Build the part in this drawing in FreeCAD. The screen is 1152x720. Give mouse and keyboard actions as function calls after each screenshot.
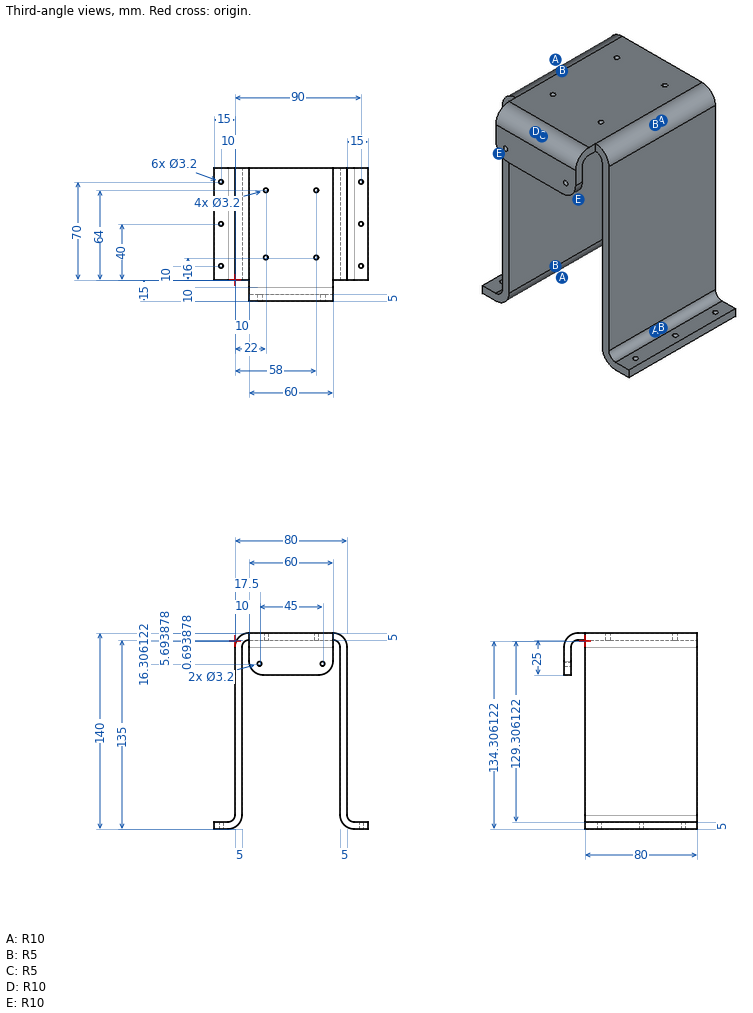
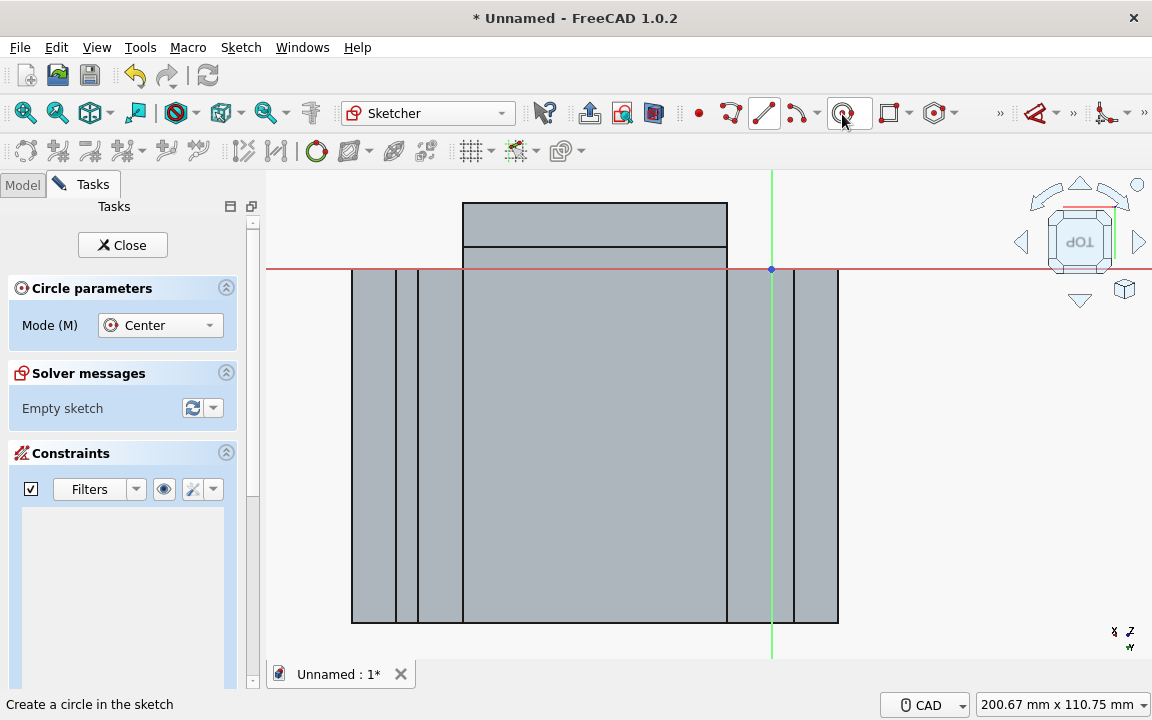
scroll(674, 552, up, 6)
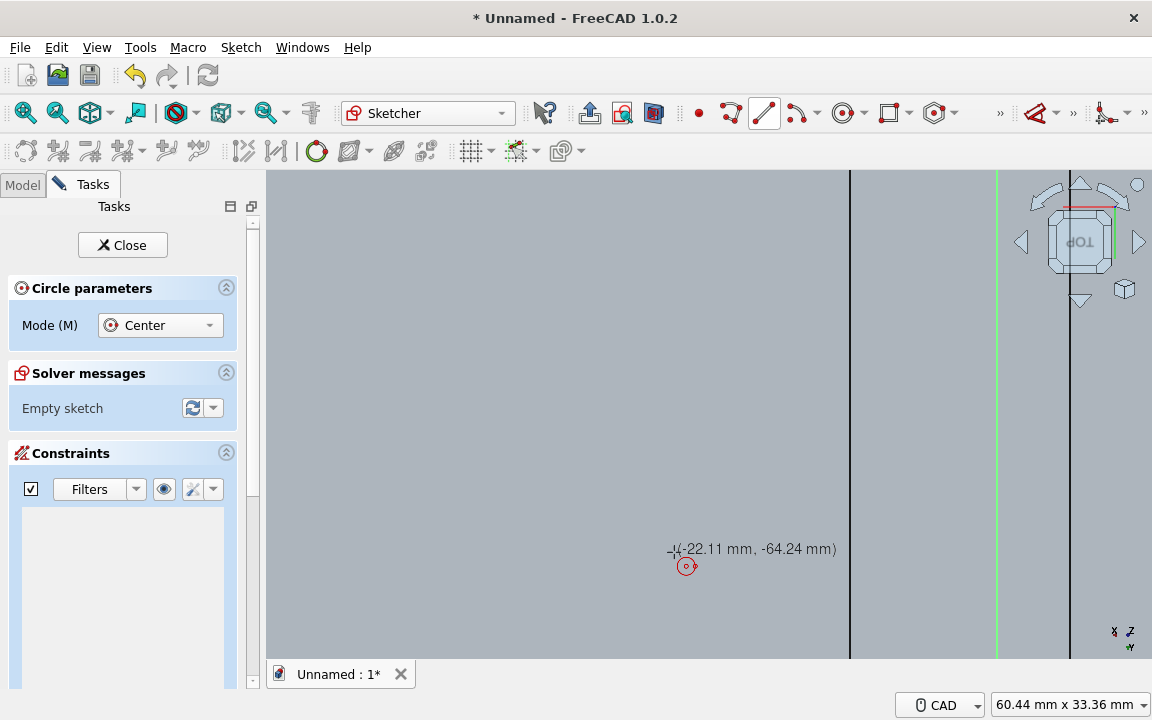
click(675, 550)
move(691, 533)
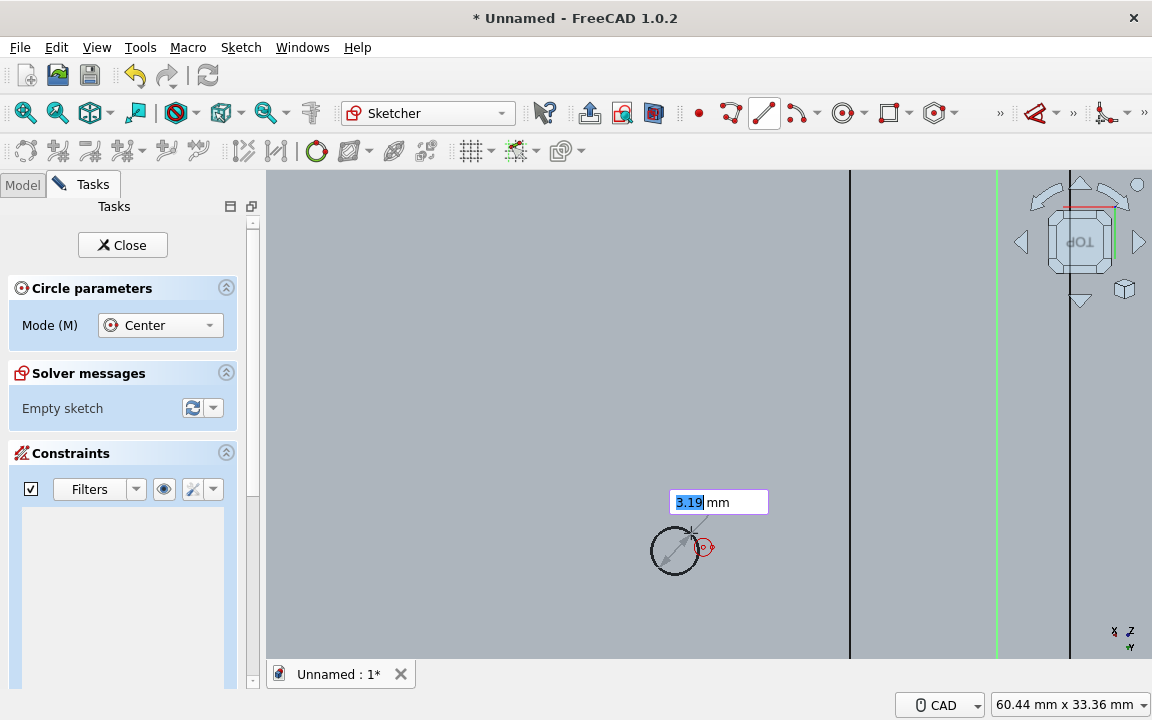
text(3.2)
key(Return)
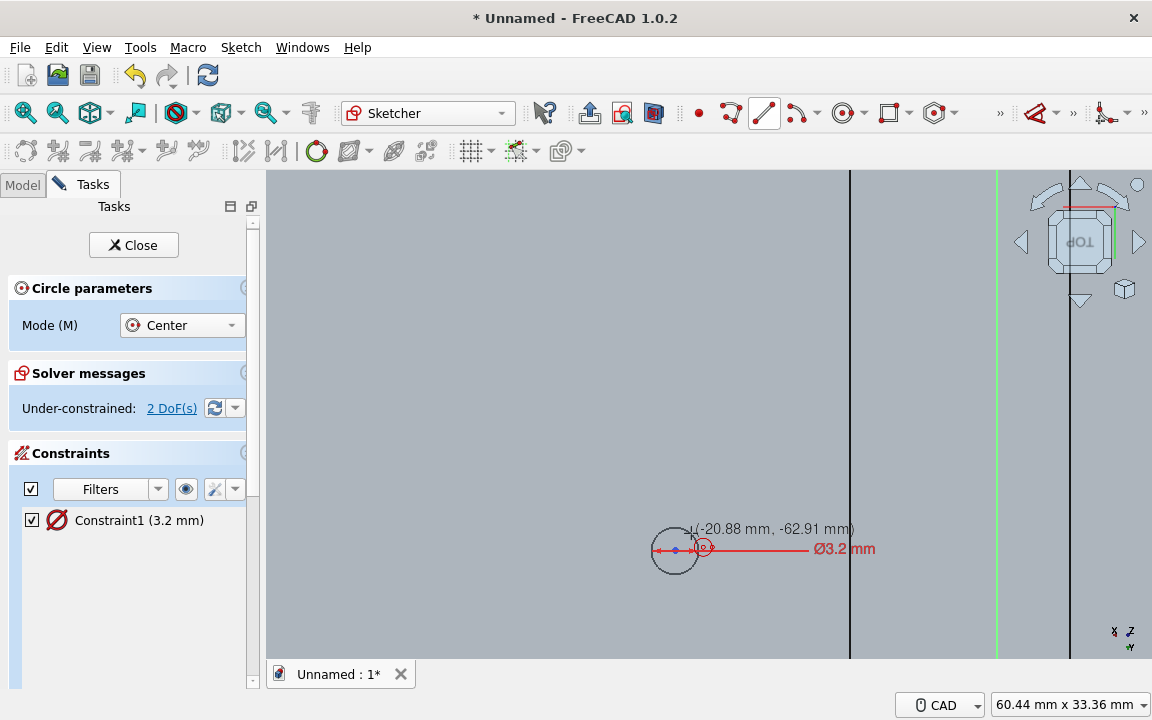
scroll(675, 553, down, 6)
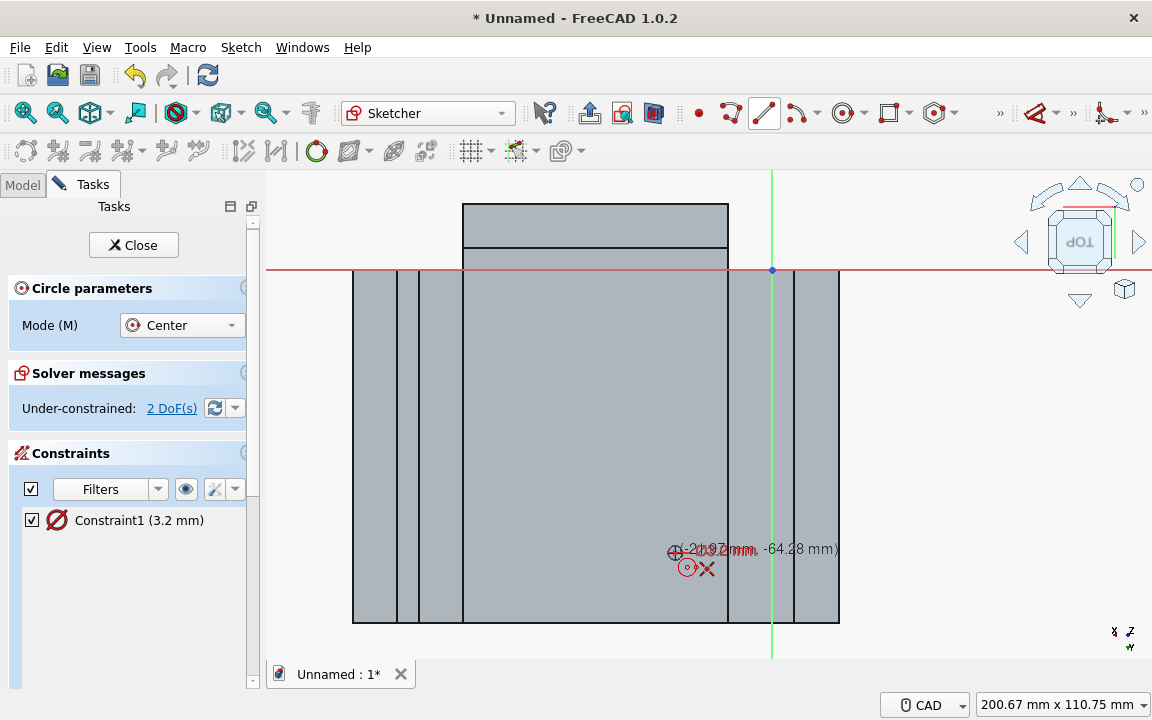
scroll(516, 553, up, 6)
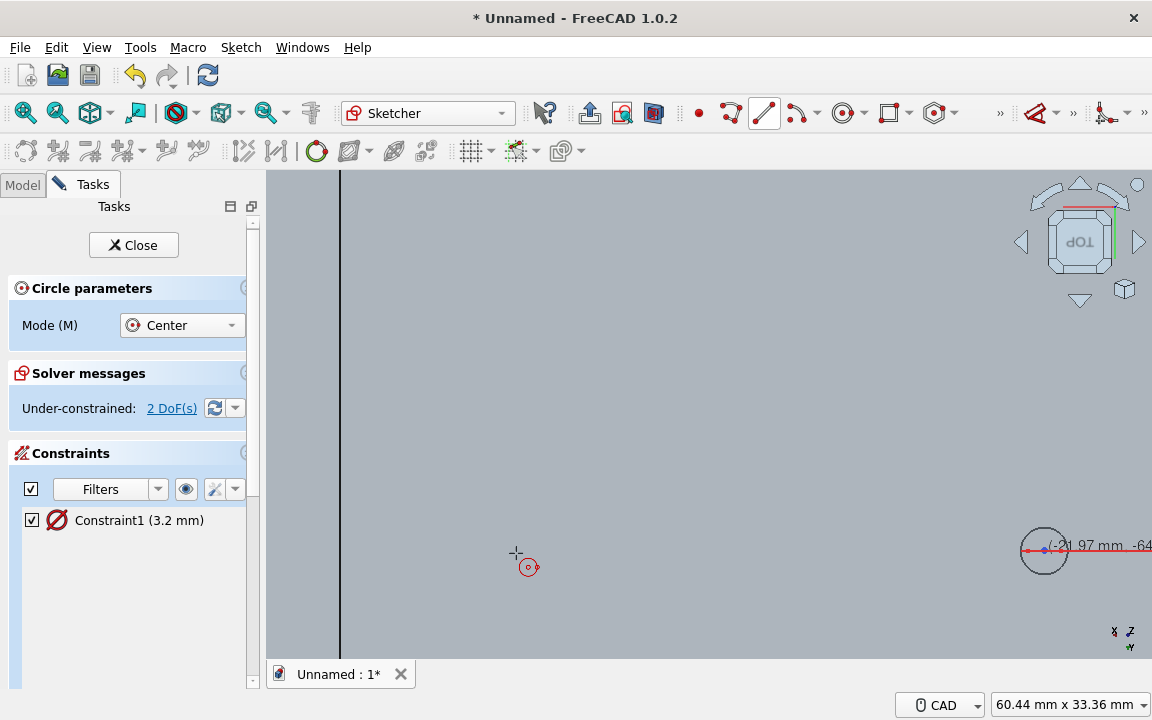
click(516, 550)
move(533, 533)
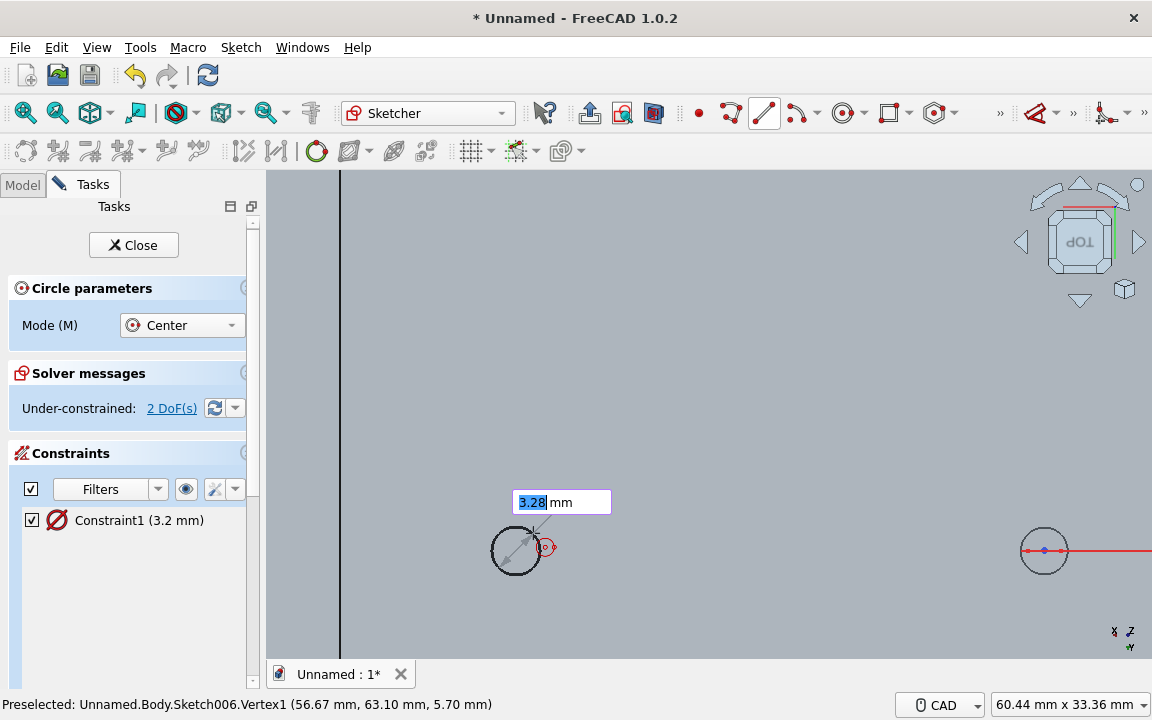
text(3.2)
key(Return)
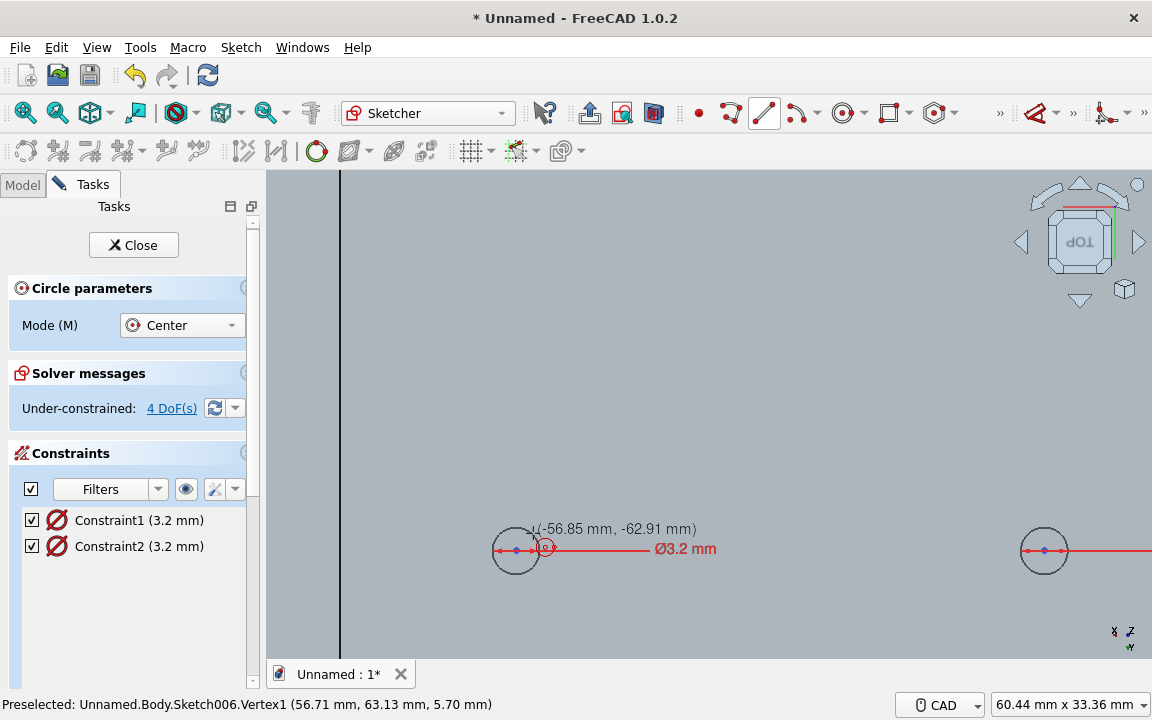
scroll(516, 553, down, 6)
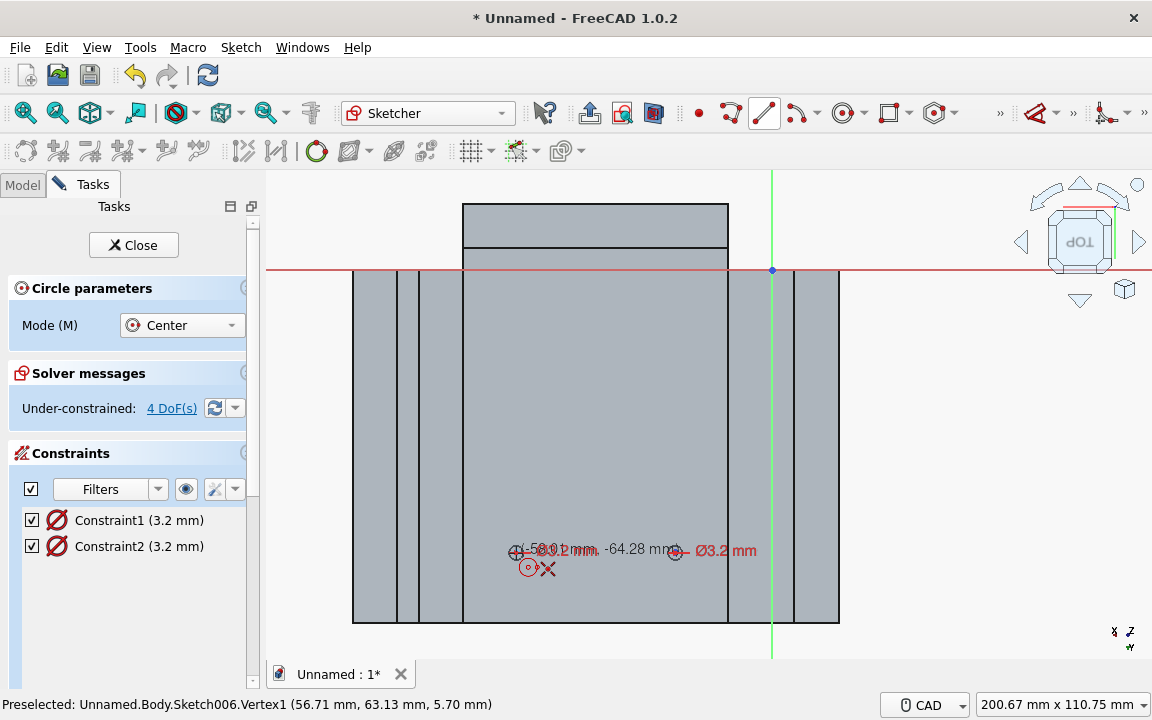
scroll(516, 341, up, 6)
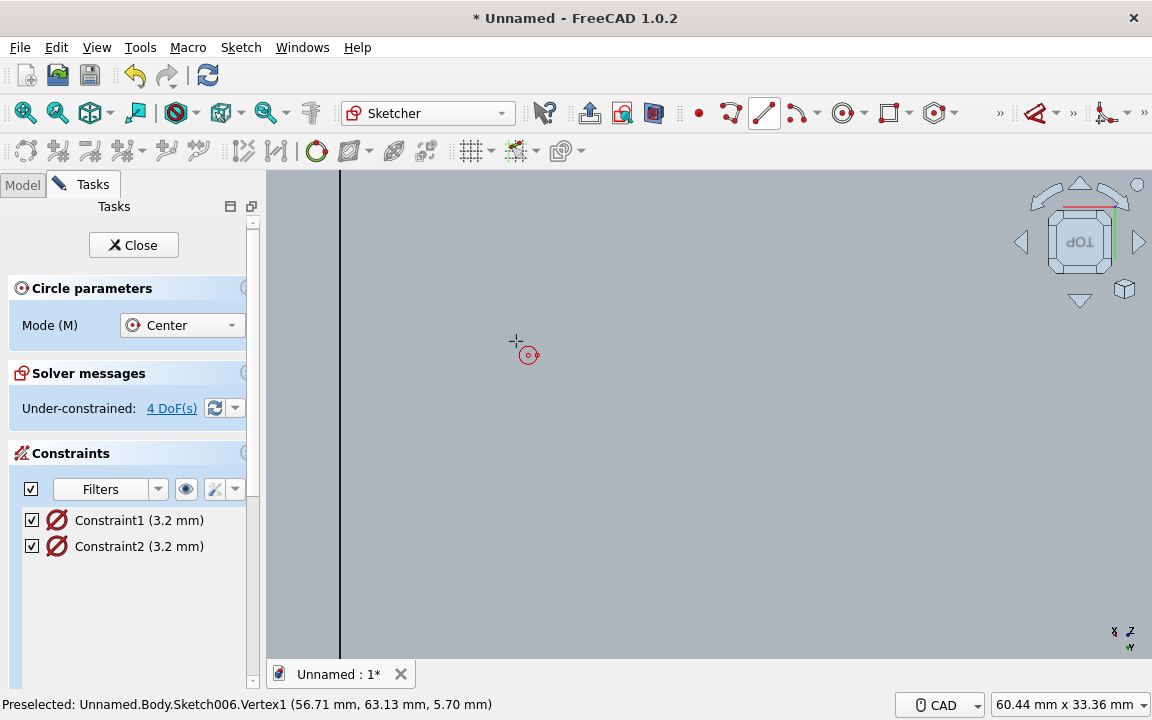
click(516, 339)
move(533, 323)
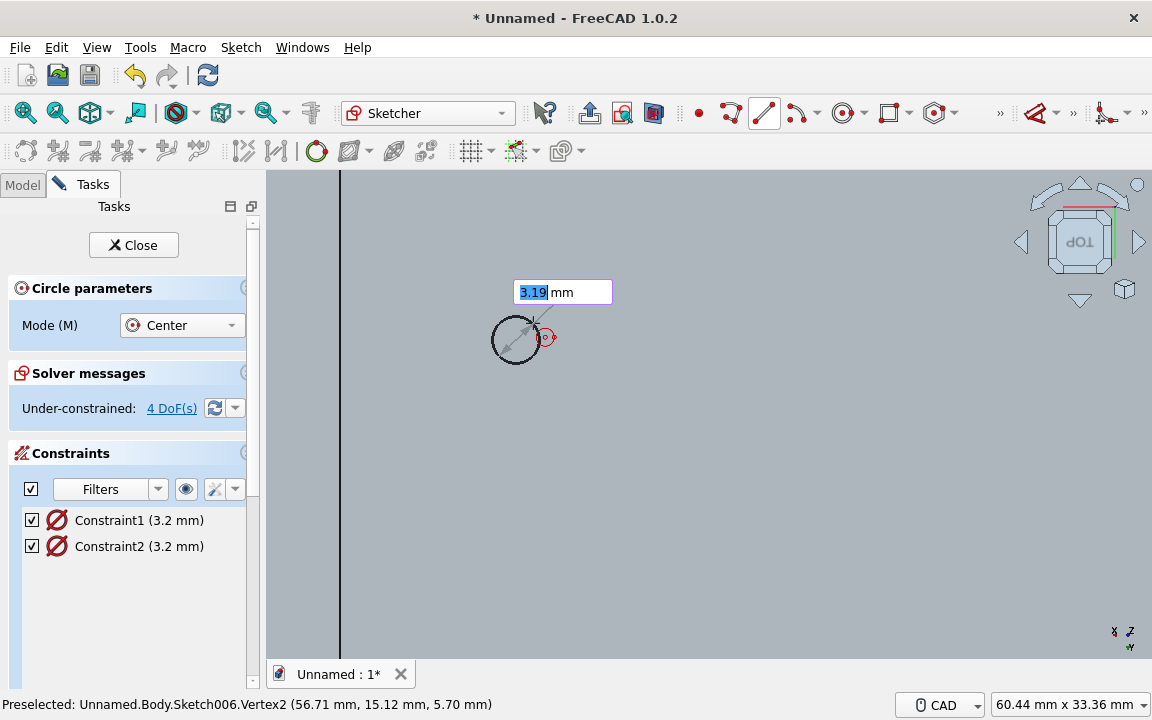
text(3.2)
key(Return)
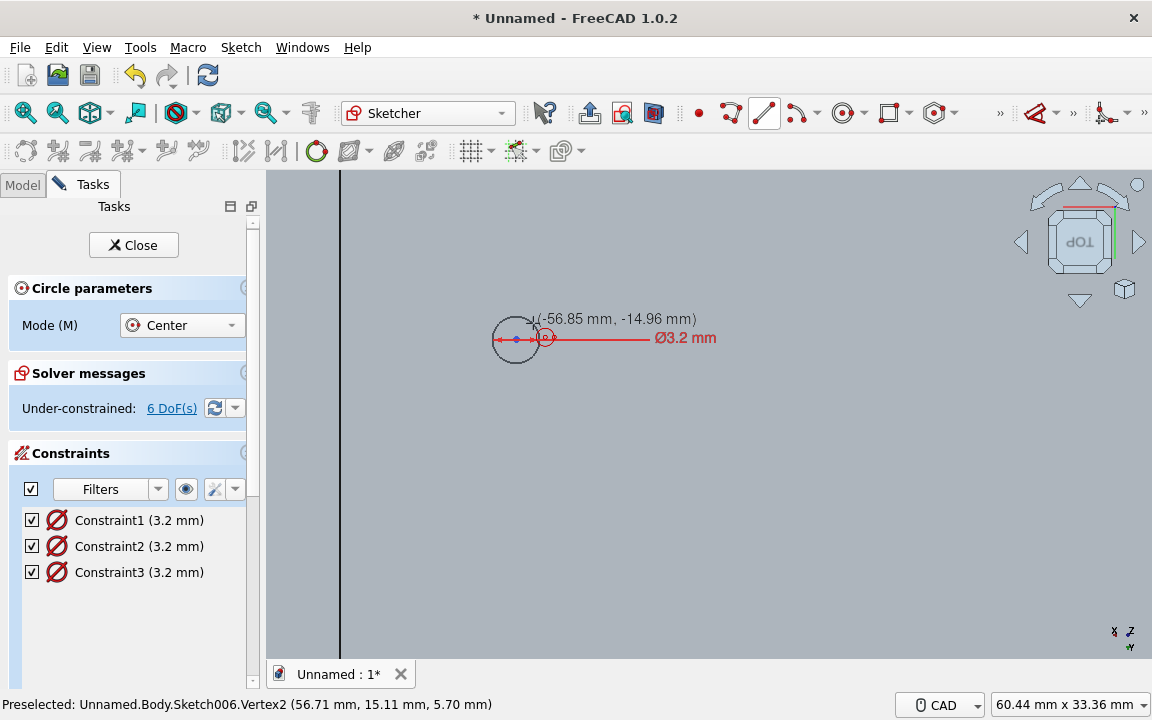
scroll(516, 341, down, 6)